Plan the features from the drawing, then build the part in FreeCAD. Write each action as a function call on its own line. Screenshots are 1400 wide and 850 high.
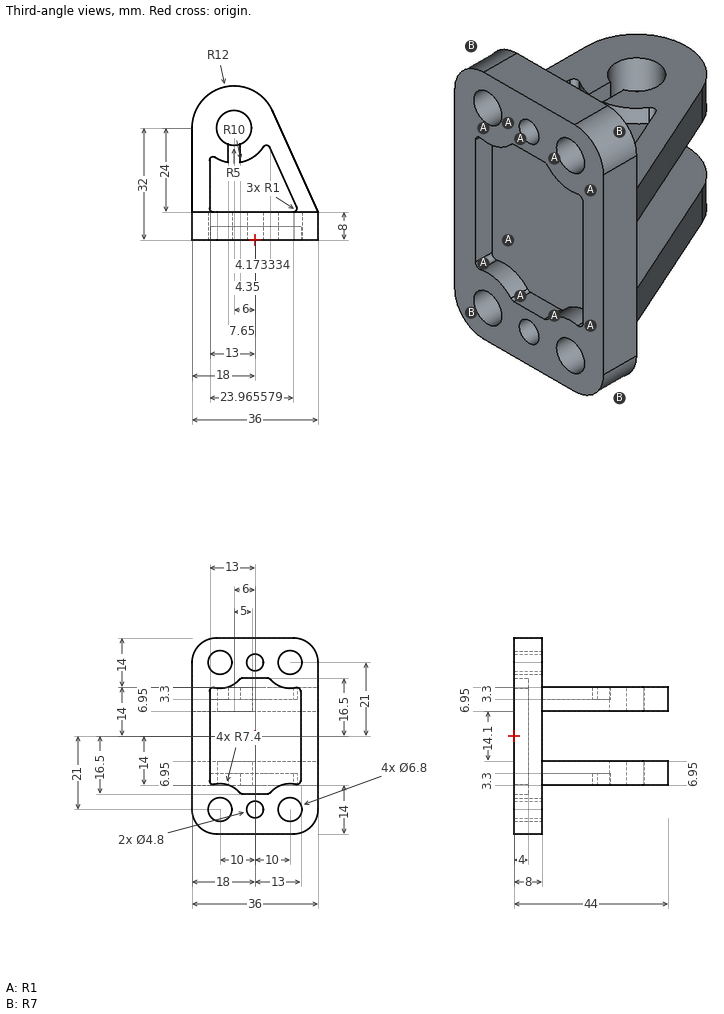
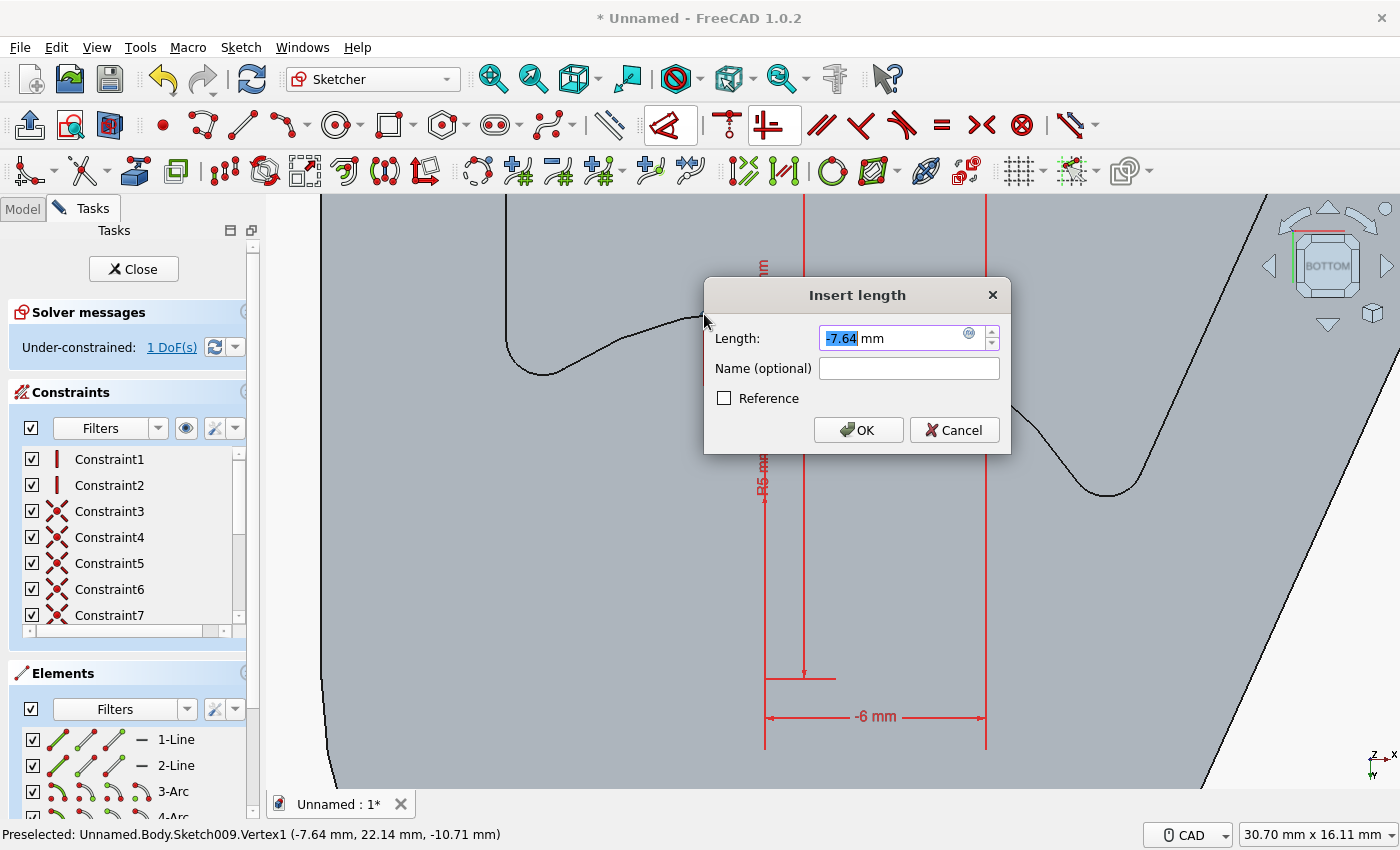
text(-7.65)
key(Return)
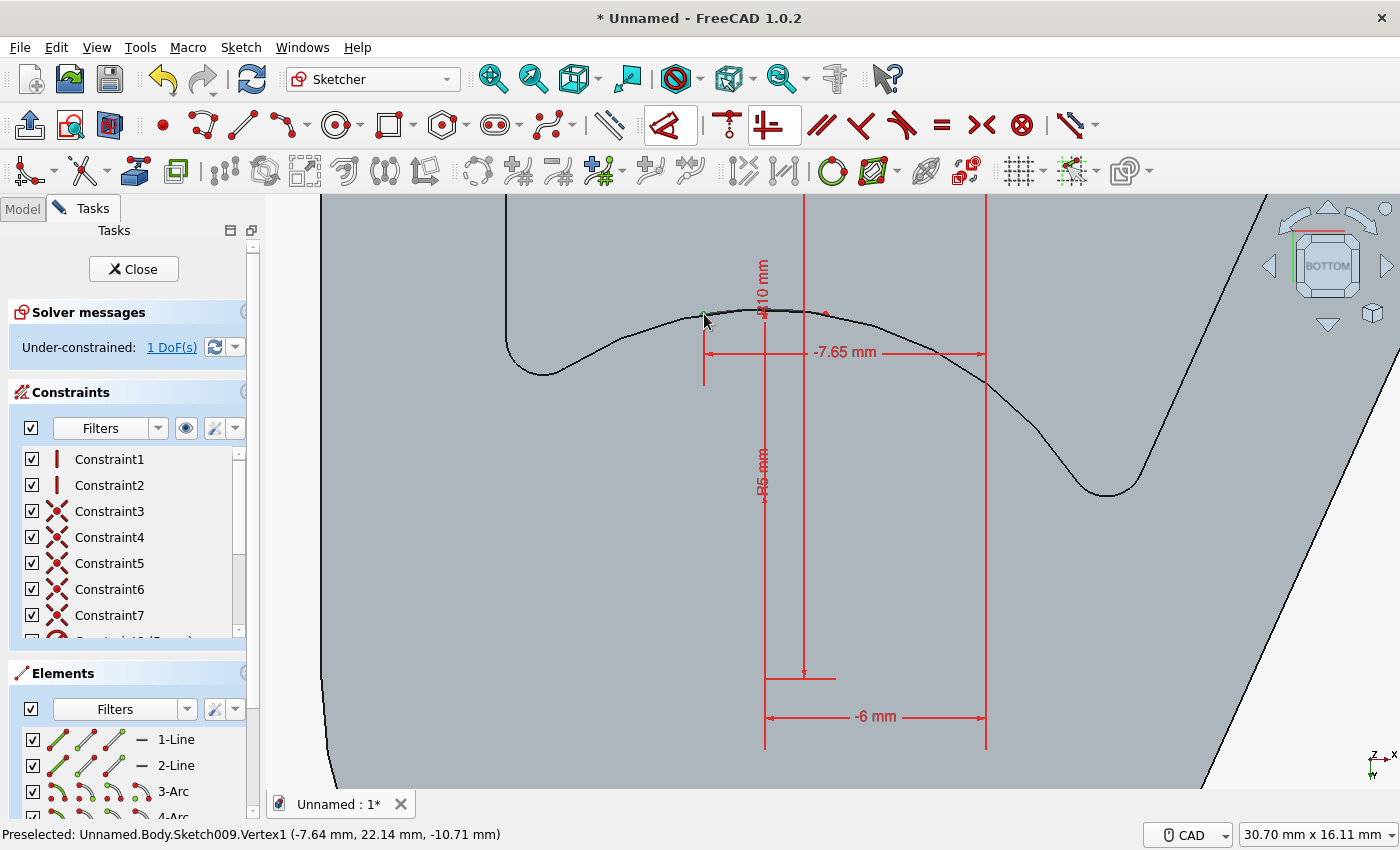
click(826, 505)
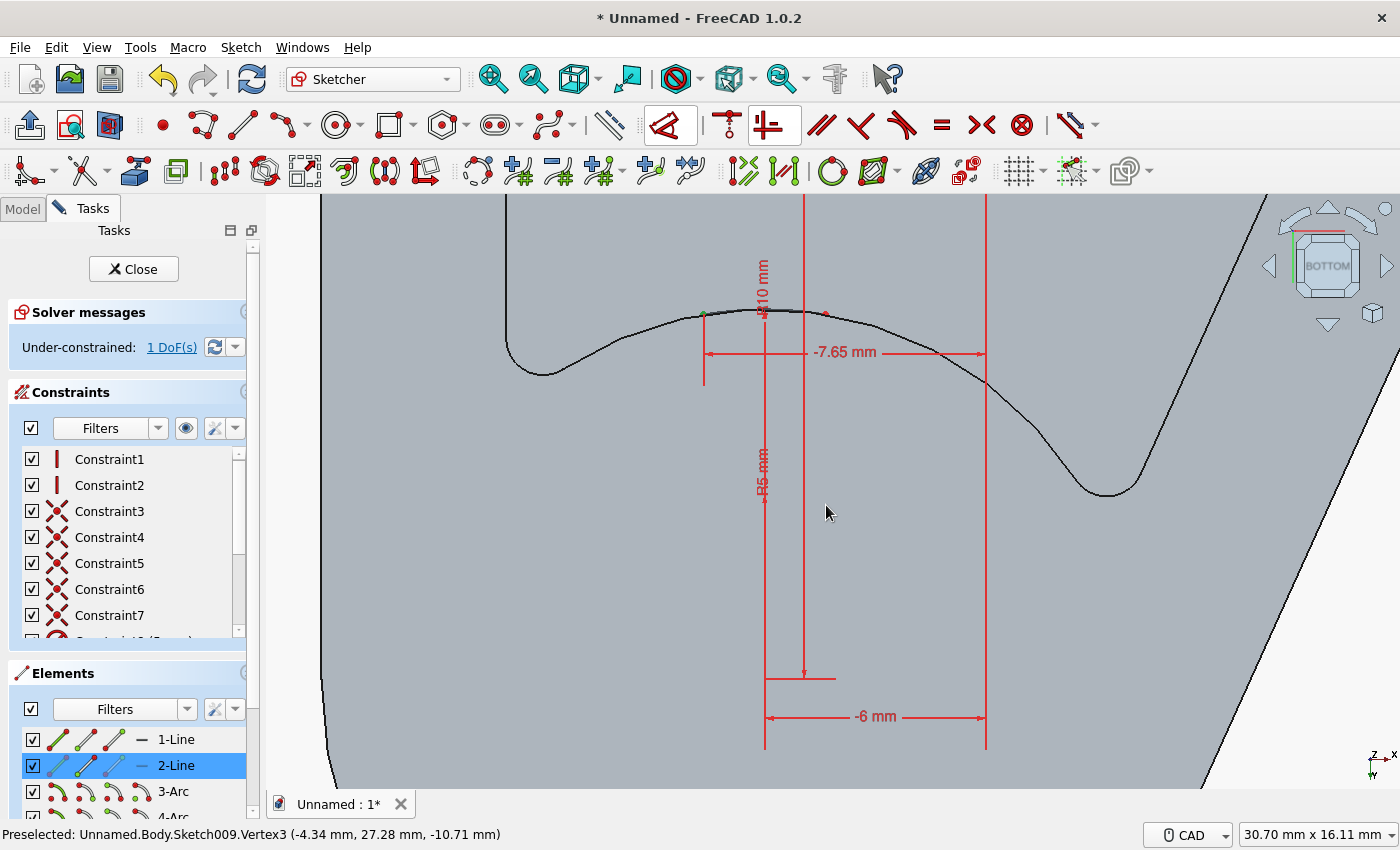
key(l)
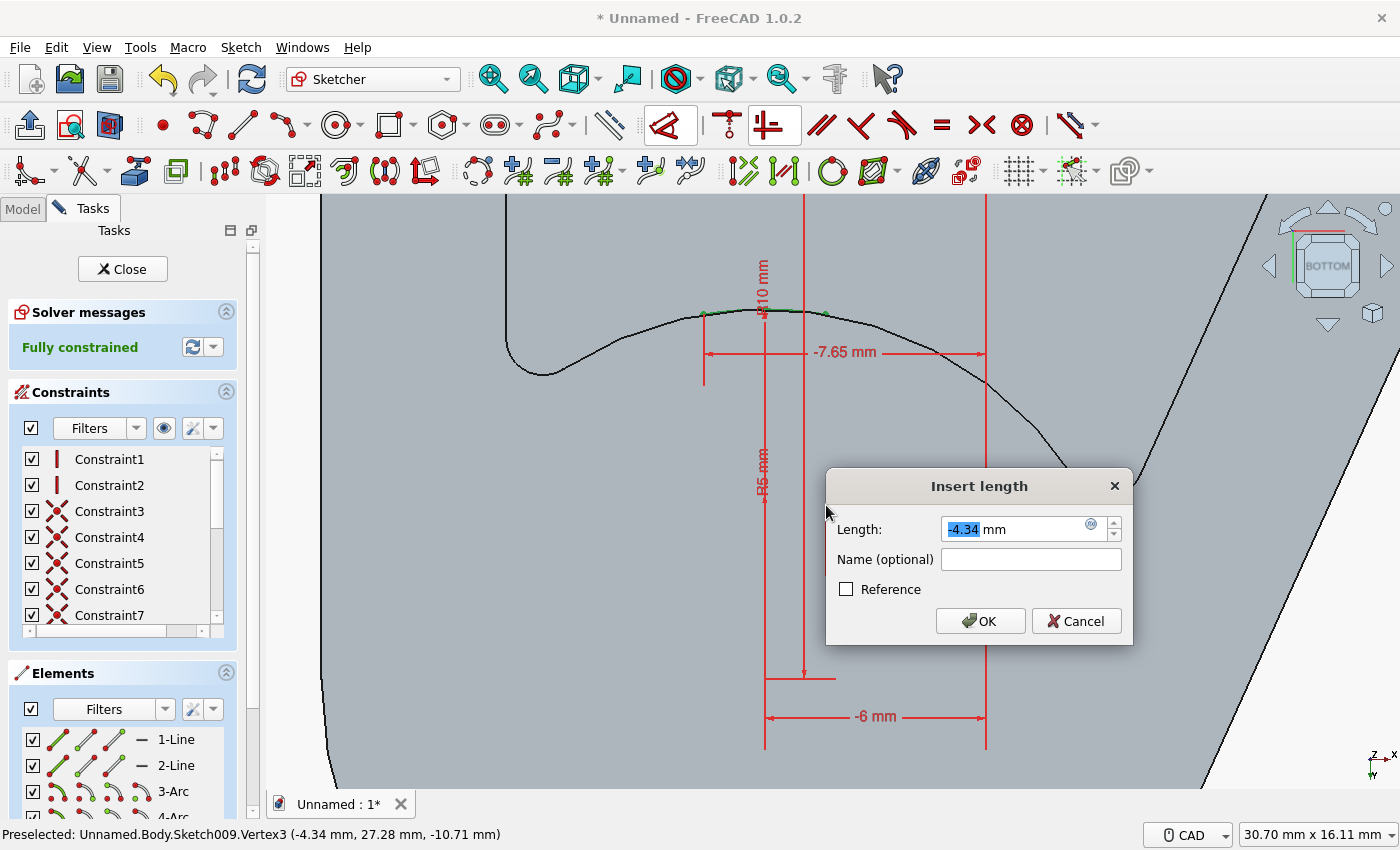
text(-4.35)
key(Return)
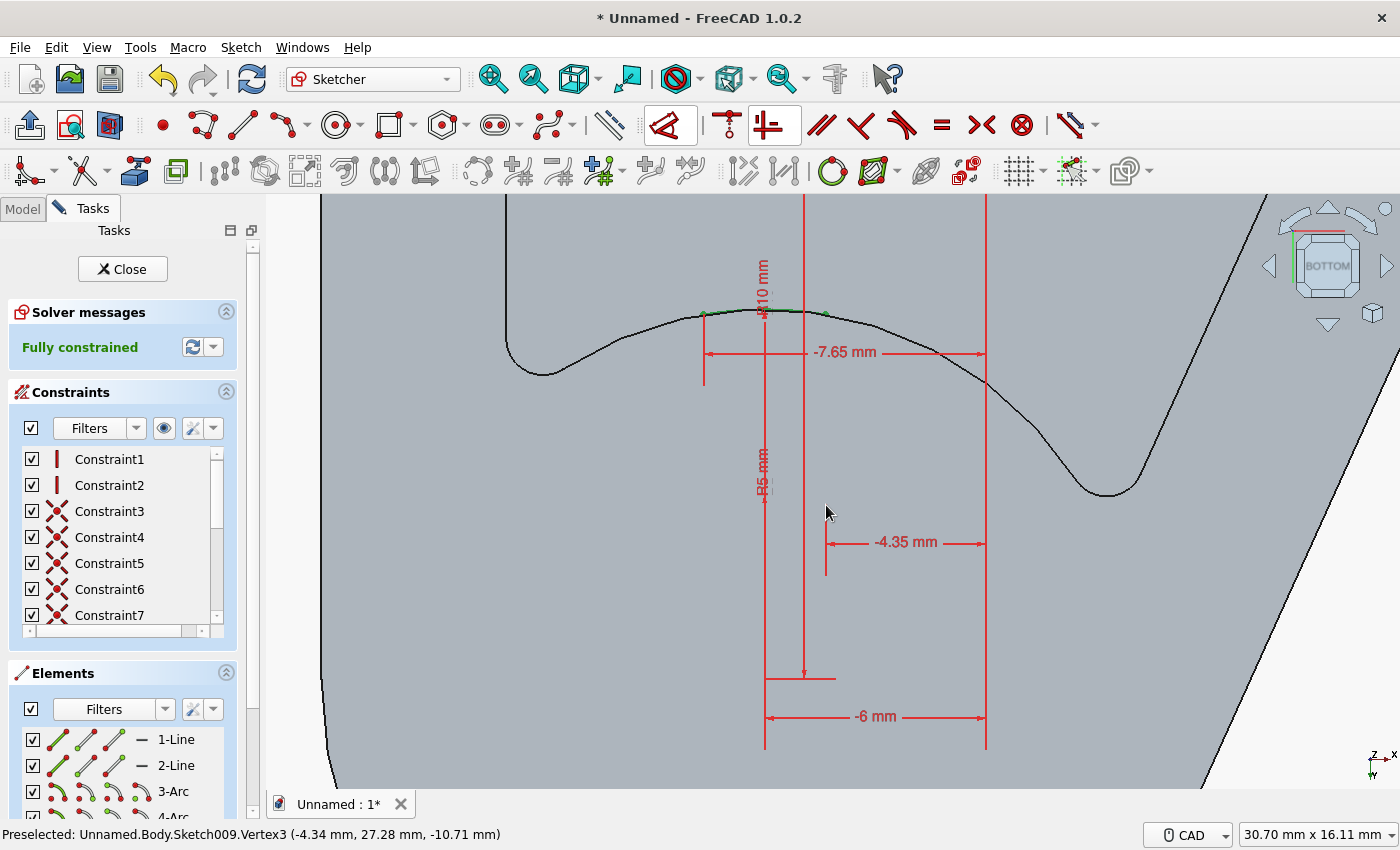
click(123, 269)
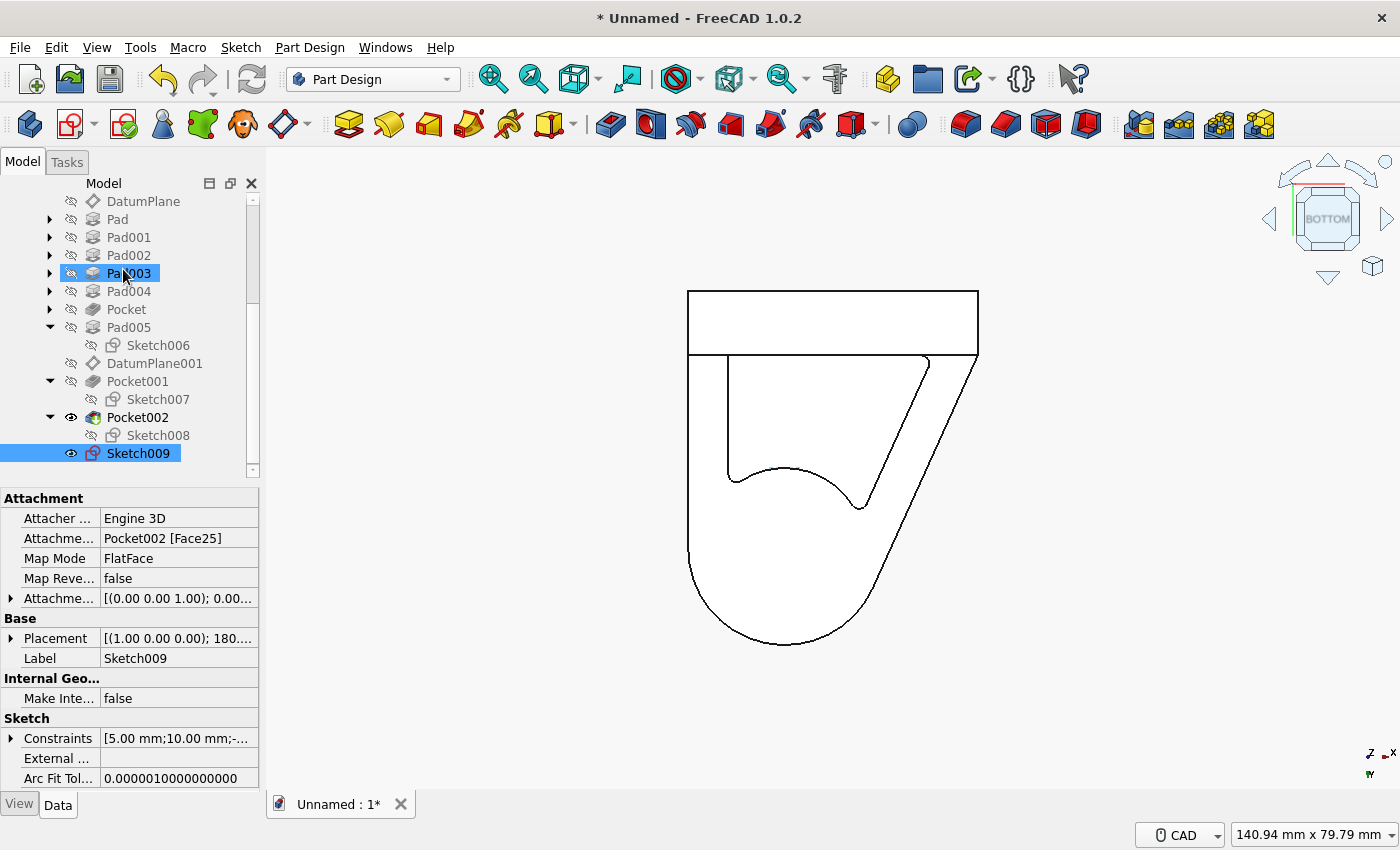
click(612, 124)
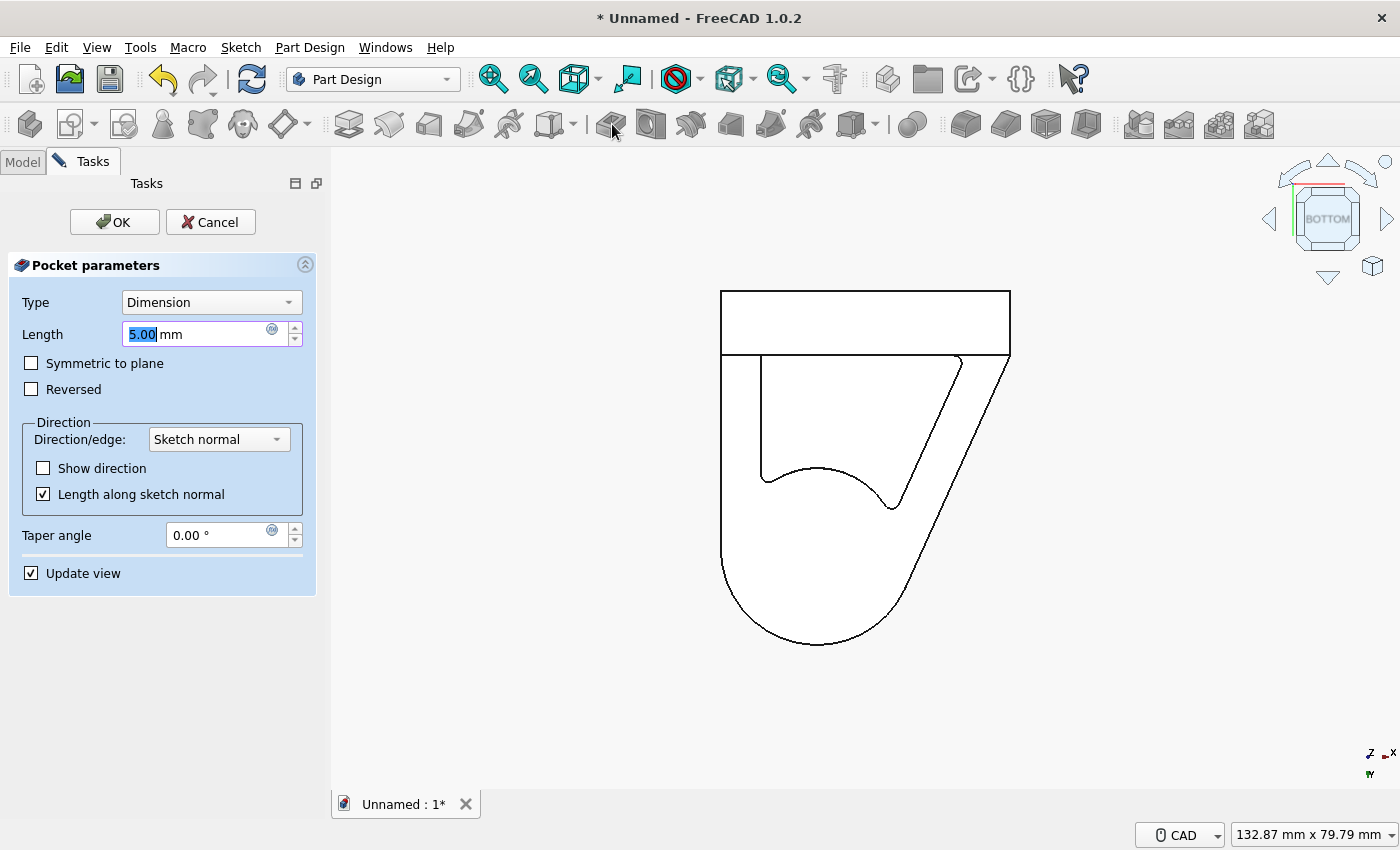
text(3.3)
key(Tab)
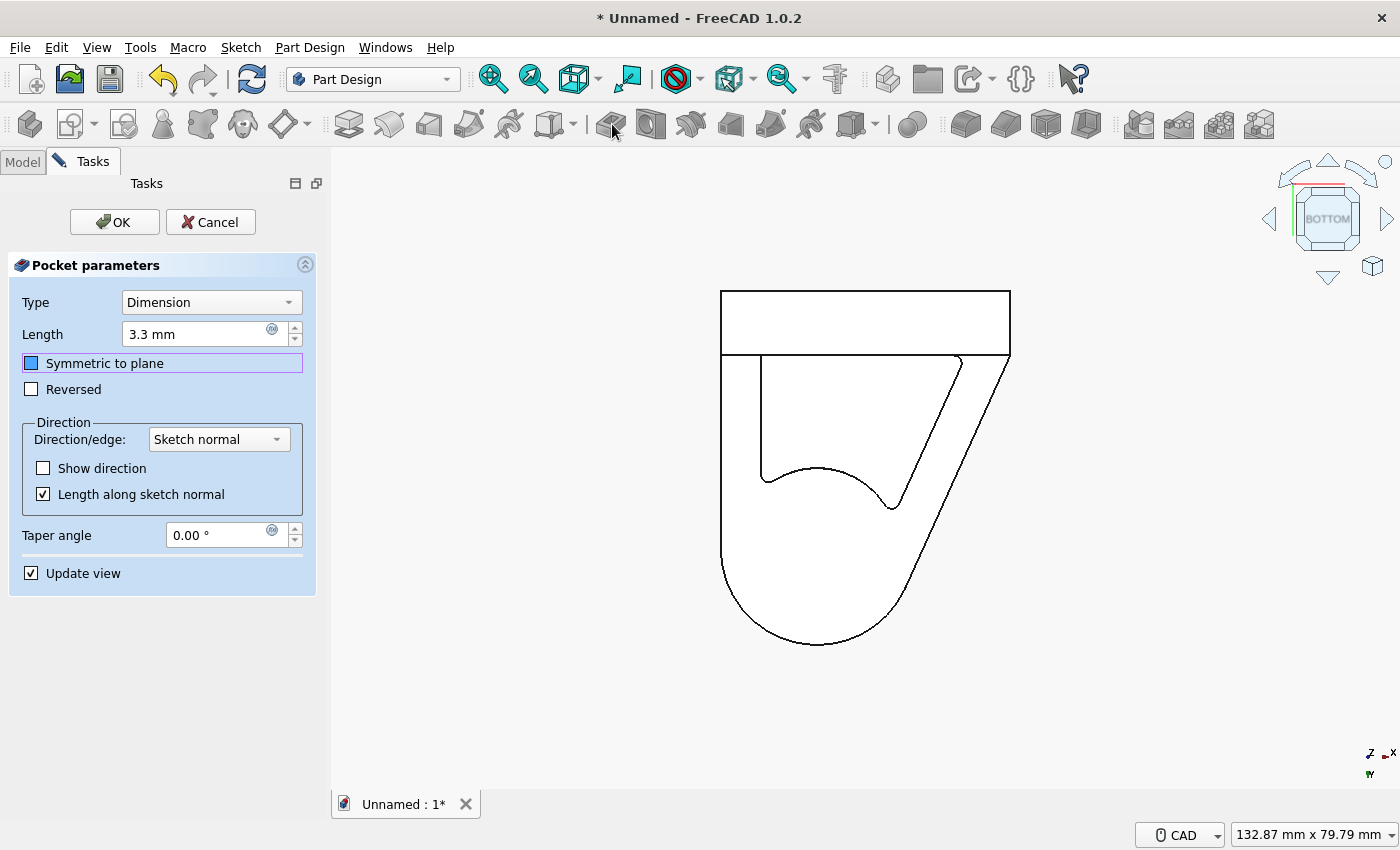
click(30, 389)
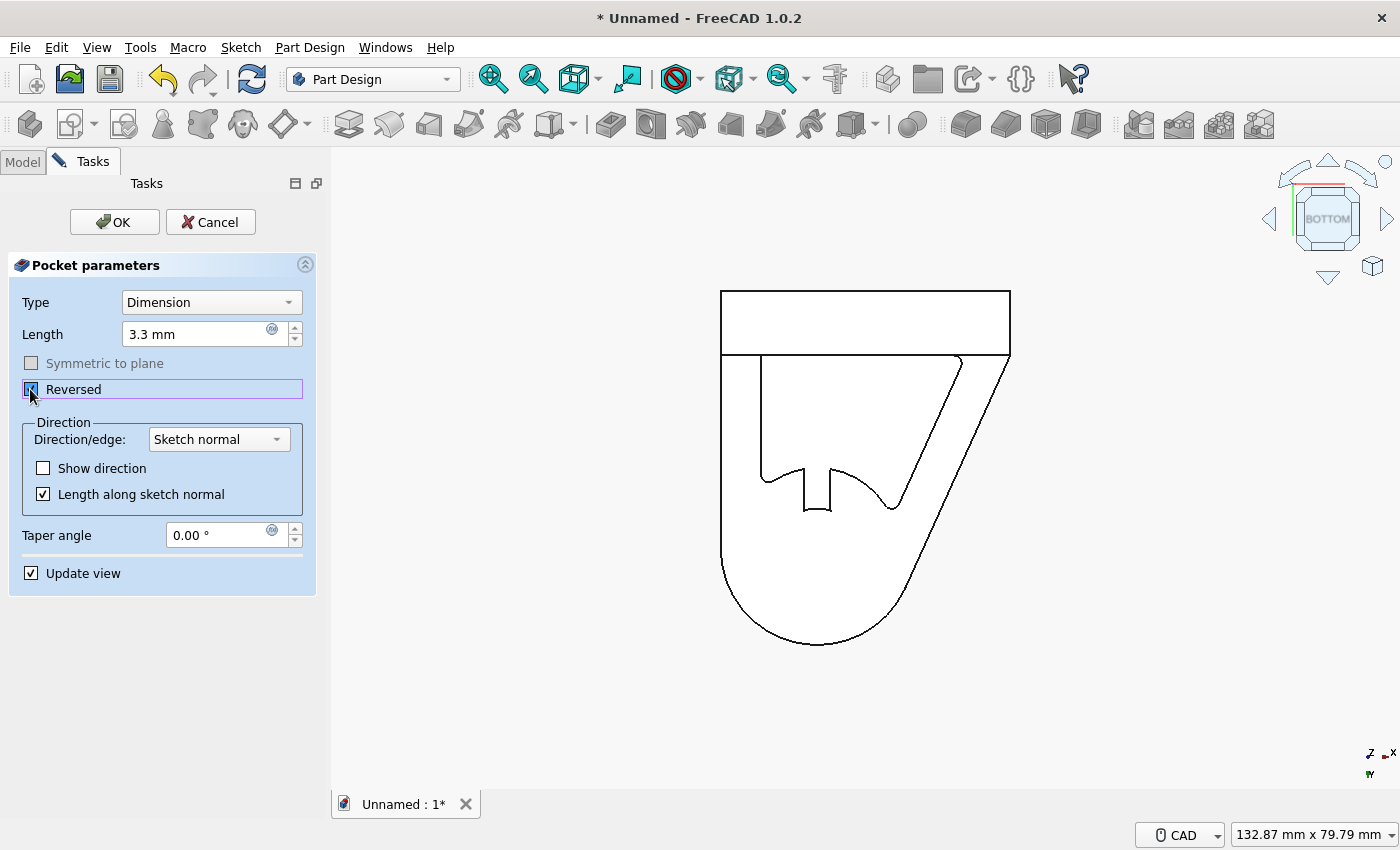
click(115, 222)